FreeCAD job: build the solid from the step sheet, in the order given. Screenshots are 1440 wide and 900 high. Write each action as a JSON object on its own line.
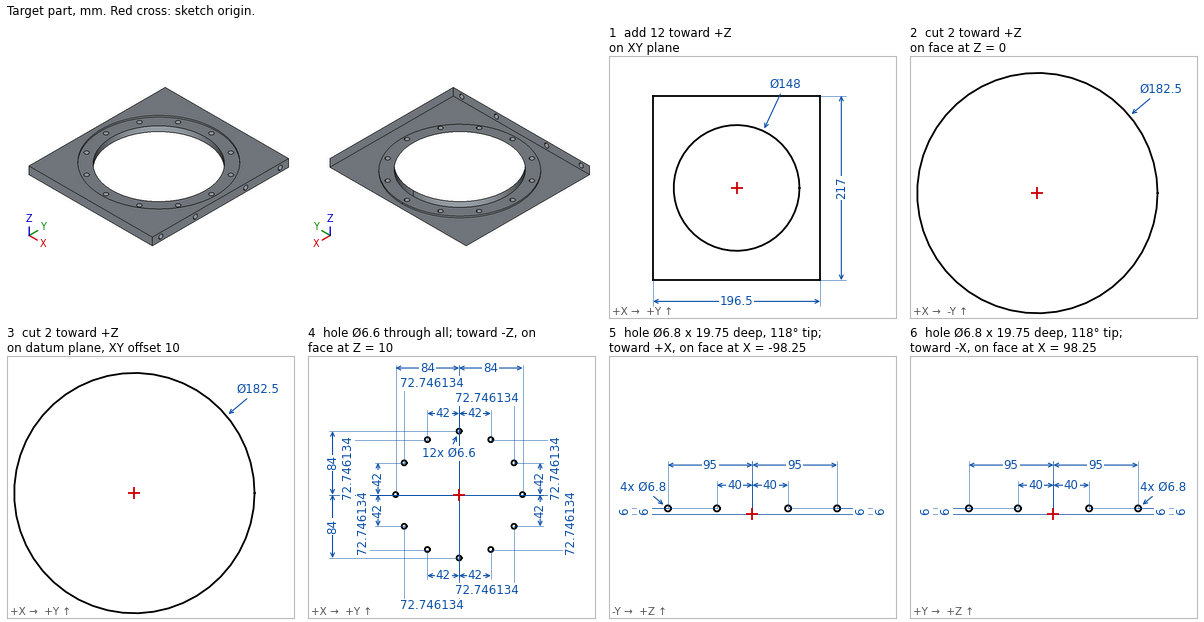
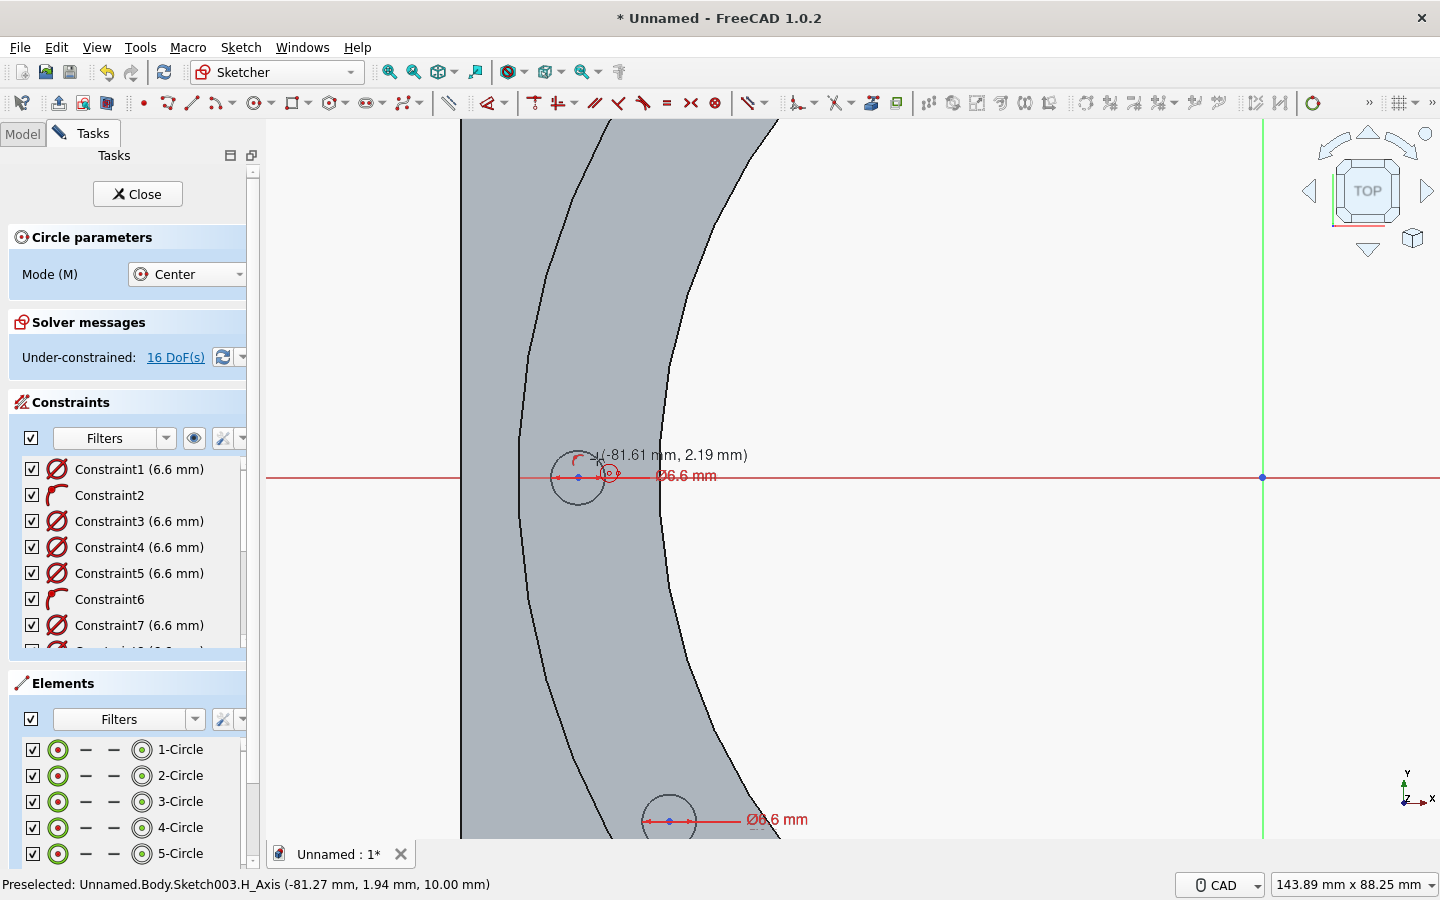
{"action": "scroll", "coordinate": [578, 480], "scroll_direction": "down", "scroll_amount": 6}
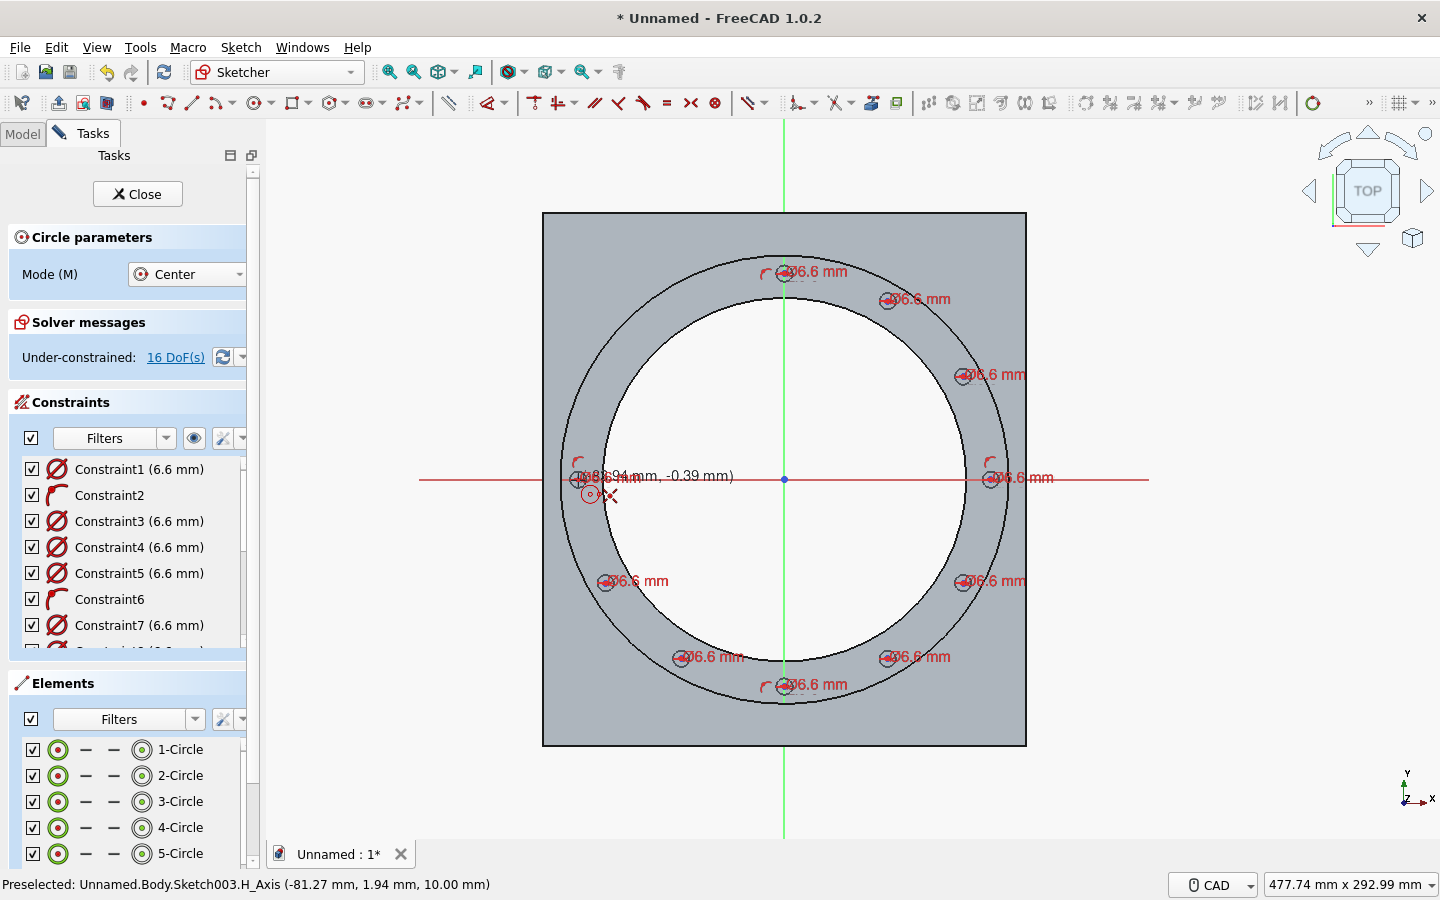
{"action": "scroll", "coordinate": [606, 376], "scroll_direction": "up", "scroll_amount": 6}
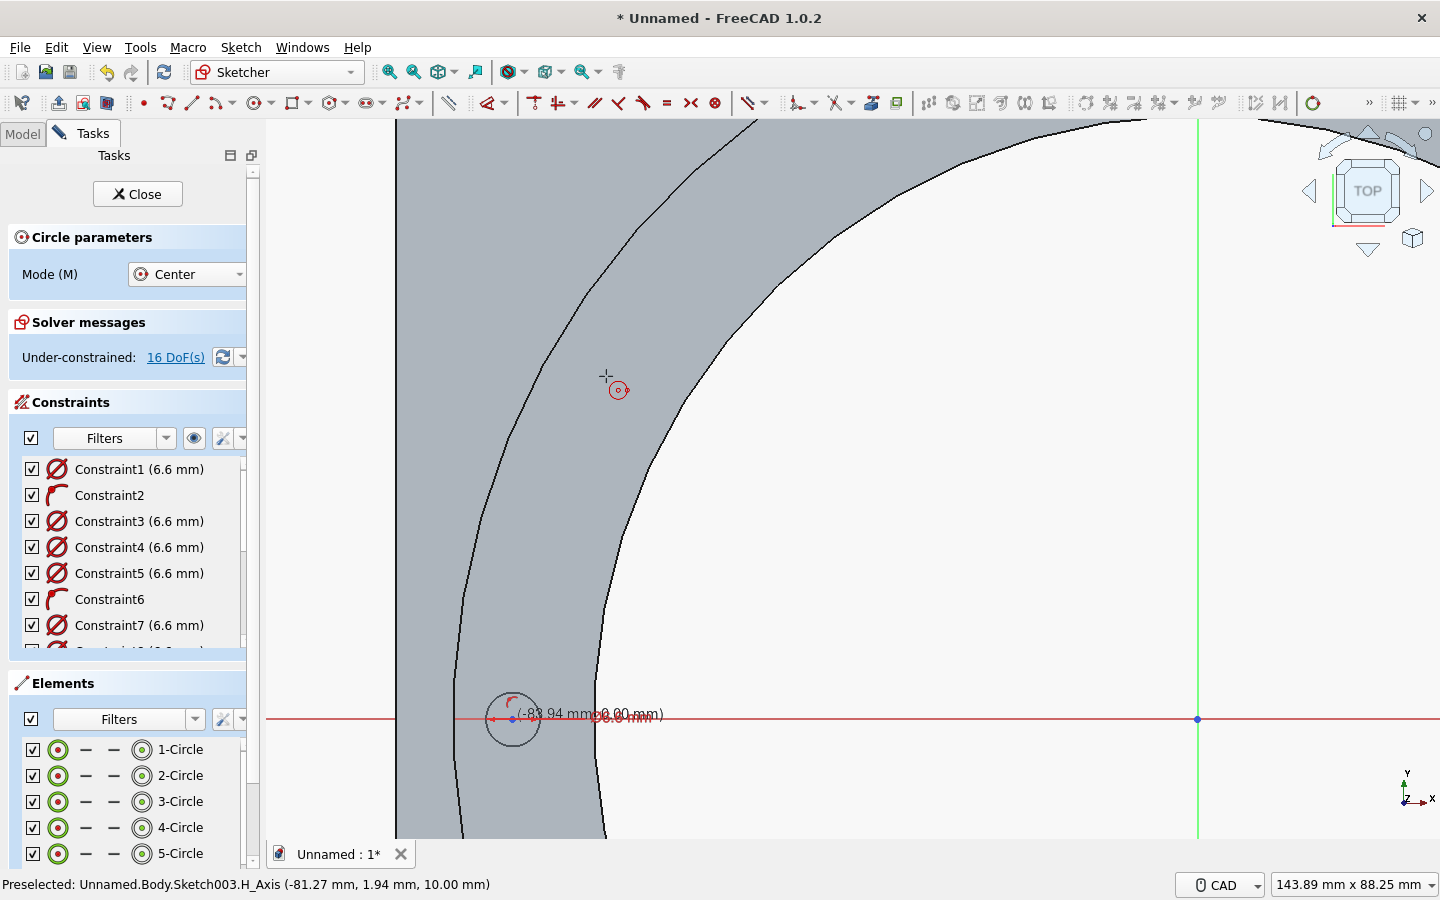
{"action": "left_click", "coordinate": [604, 377]}
{"action": "mouse_move", "coordinate": [623, 358]}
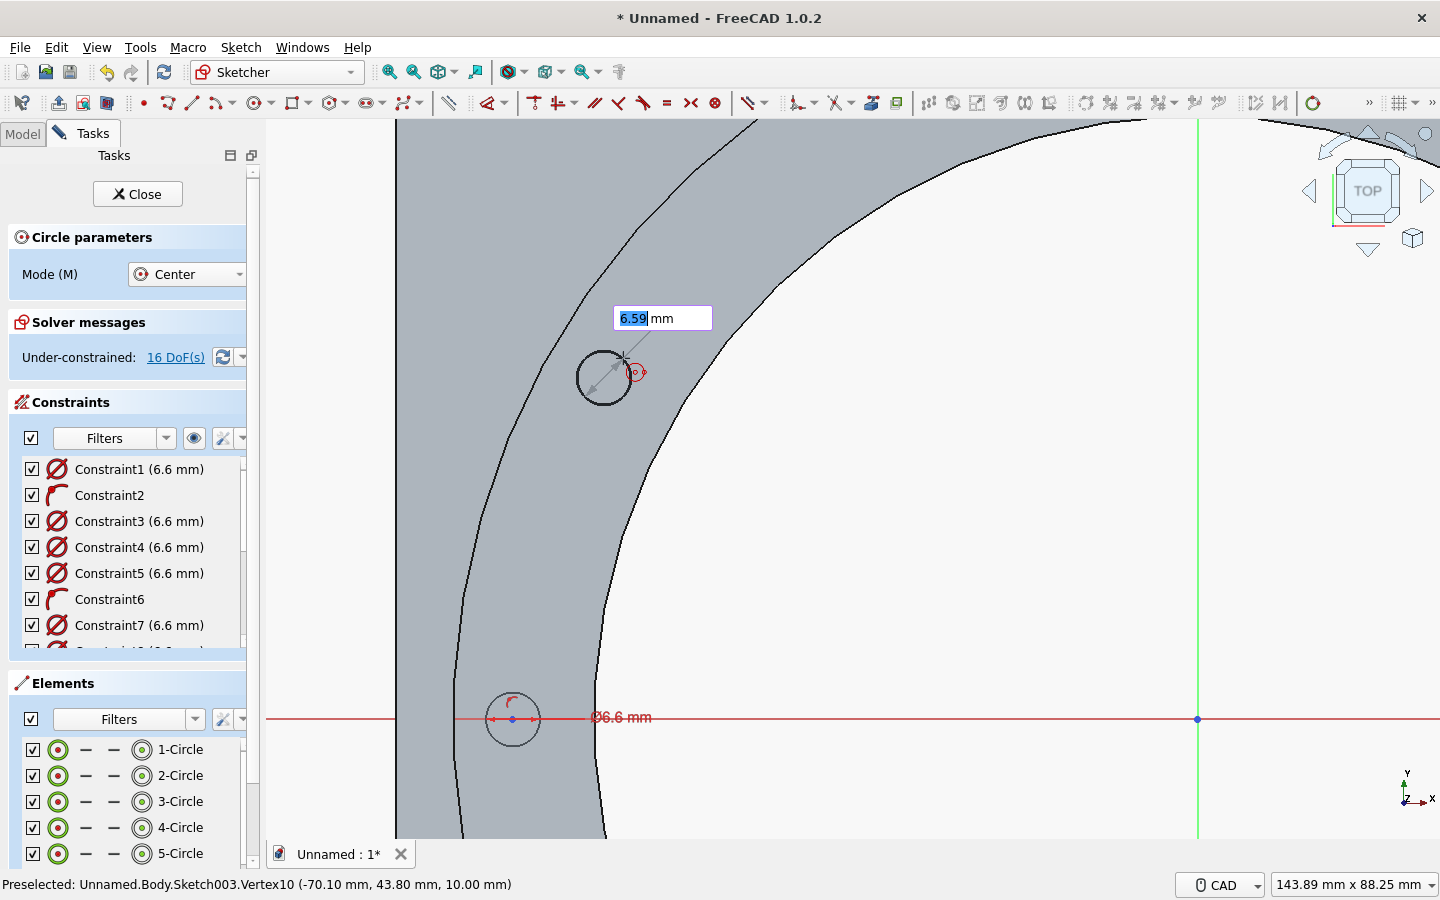
{"action": "type", "text": "6.6"}
{"action": "key", "text": "Return"}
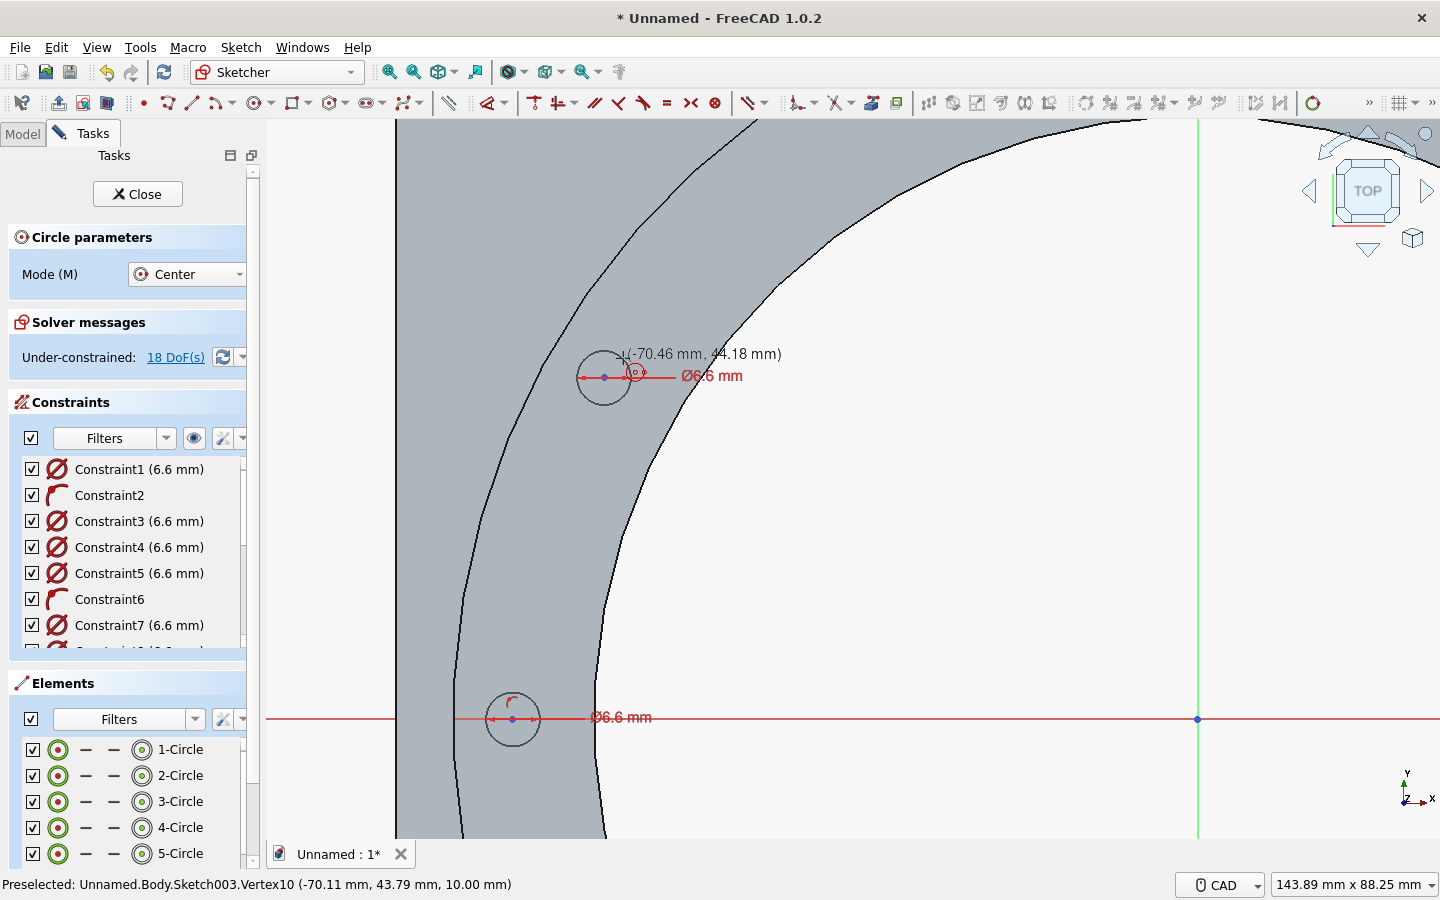
{"action": "scroll", "coordinate": [606, 375], "scroll_direction": "down", "scroll_amount": 6}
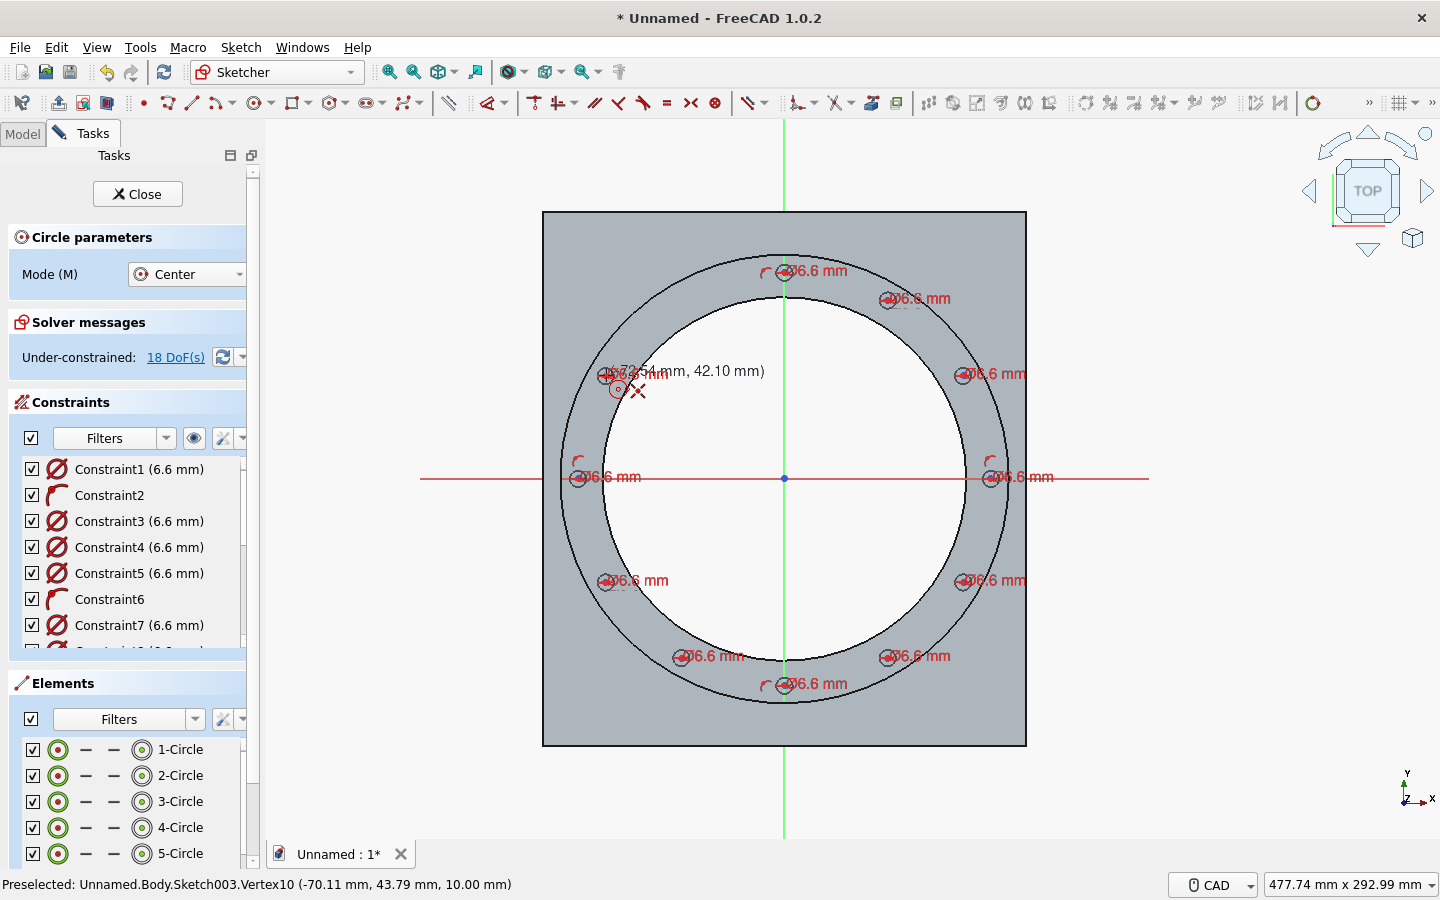
{"action": "scroll", "coordinate": [681, 300], "scroll_direction": "up", "scroll_amount": 6}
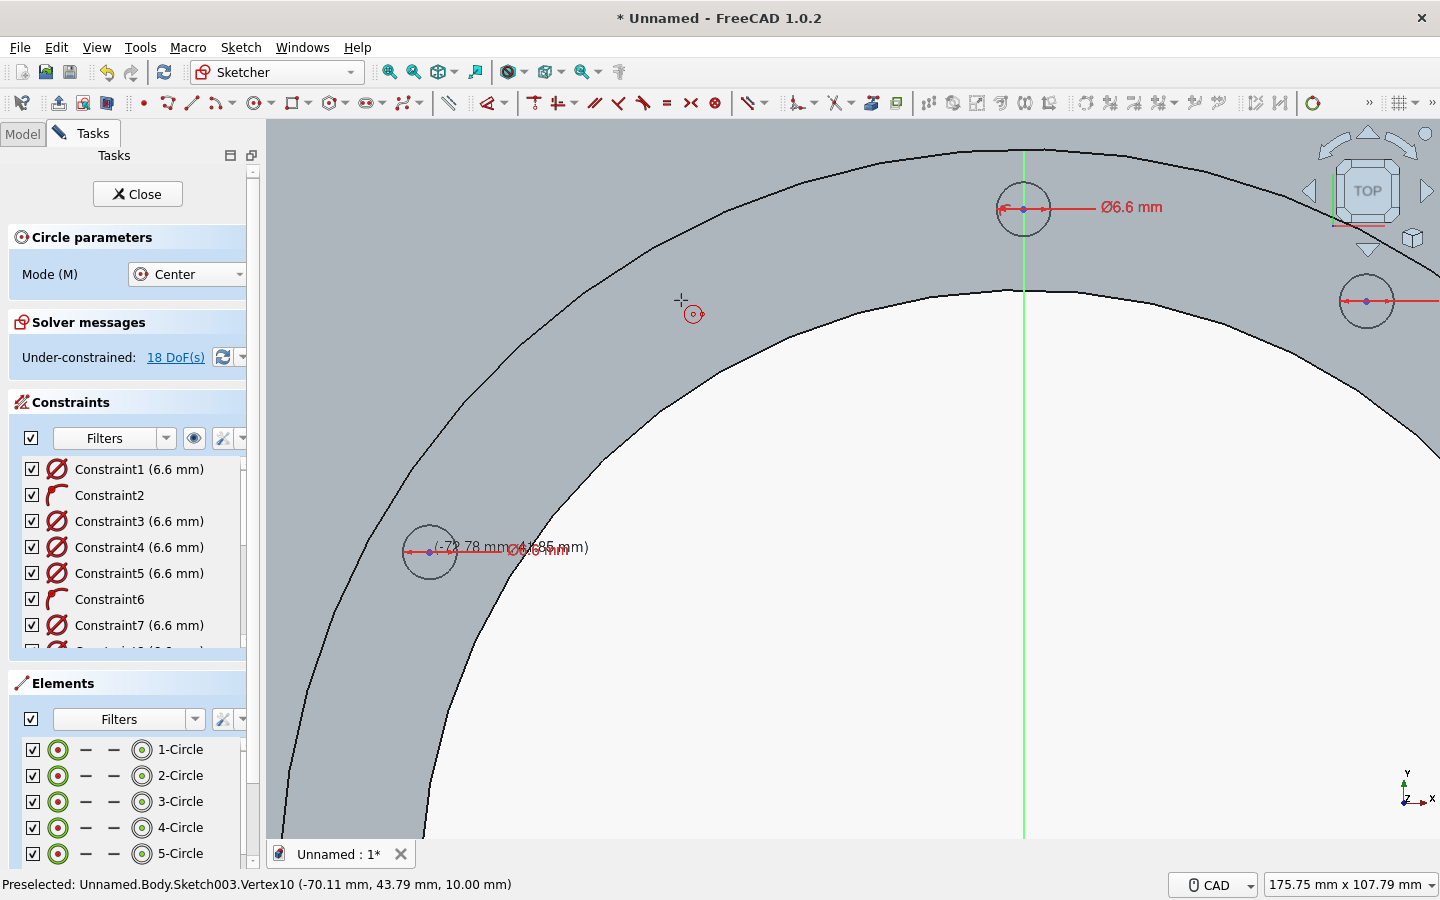
{"action": "left_click", "coordinate": [681, 300]}
{"action": "mouse_move", "coordinate": [700, 281]}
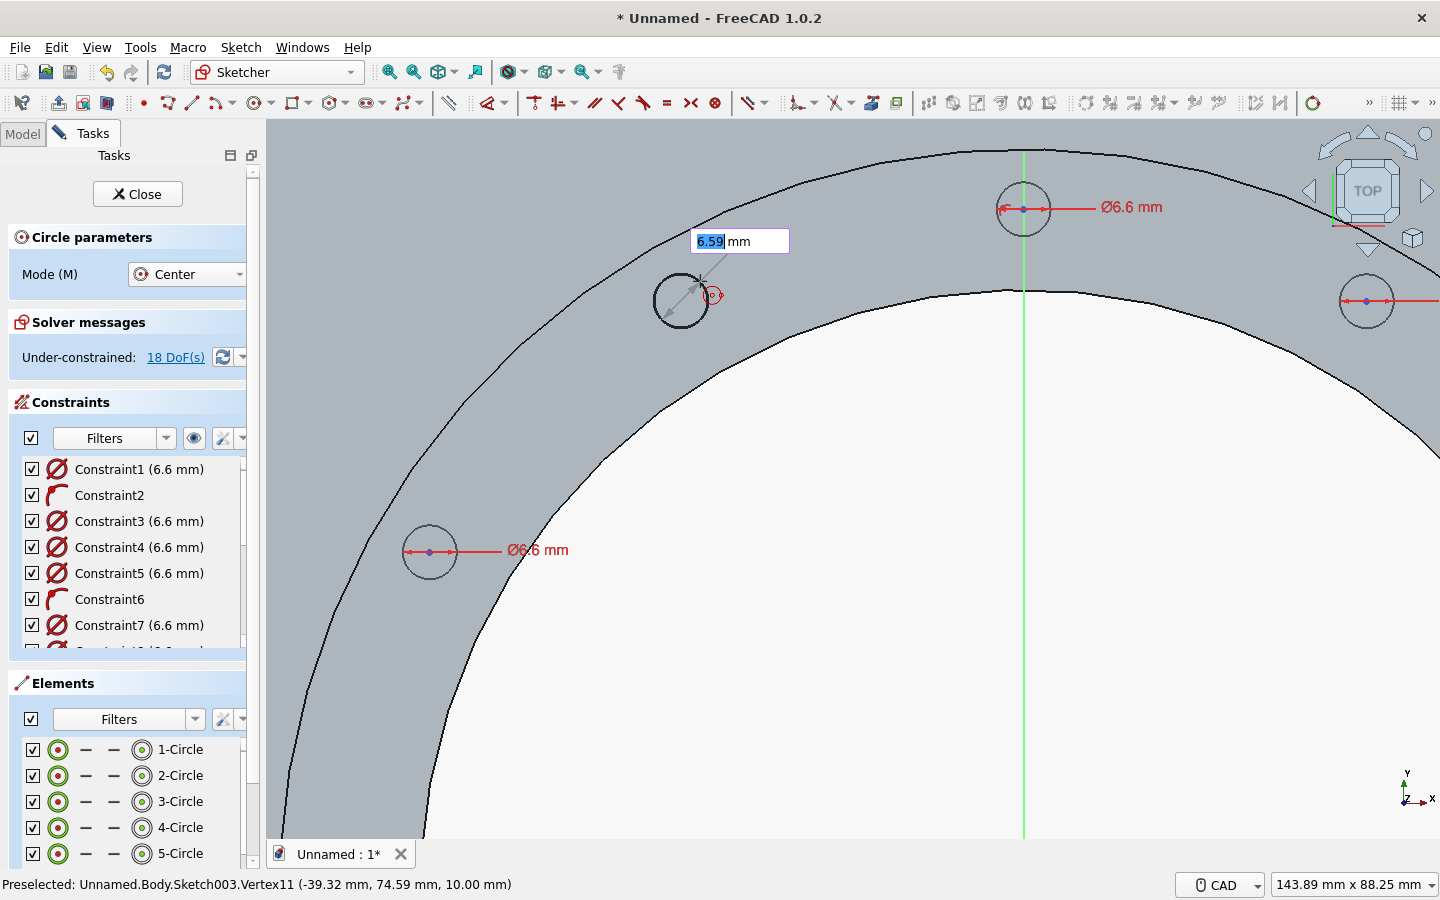
{"action": "type", "text": "6.6"}
{"action": "key", "text": "Return"}
{"action": "key", "text": "Escape"}